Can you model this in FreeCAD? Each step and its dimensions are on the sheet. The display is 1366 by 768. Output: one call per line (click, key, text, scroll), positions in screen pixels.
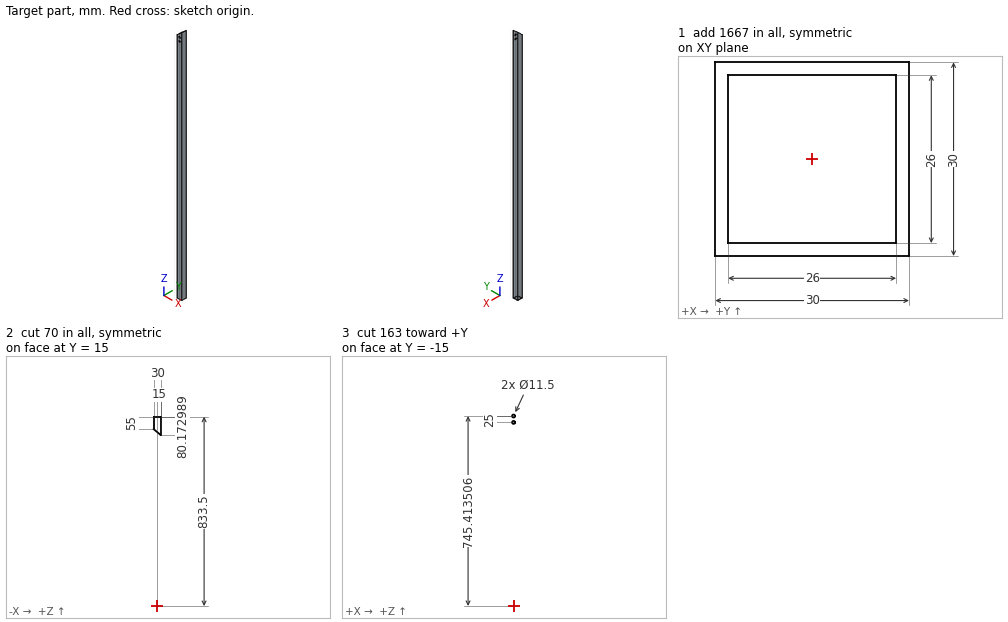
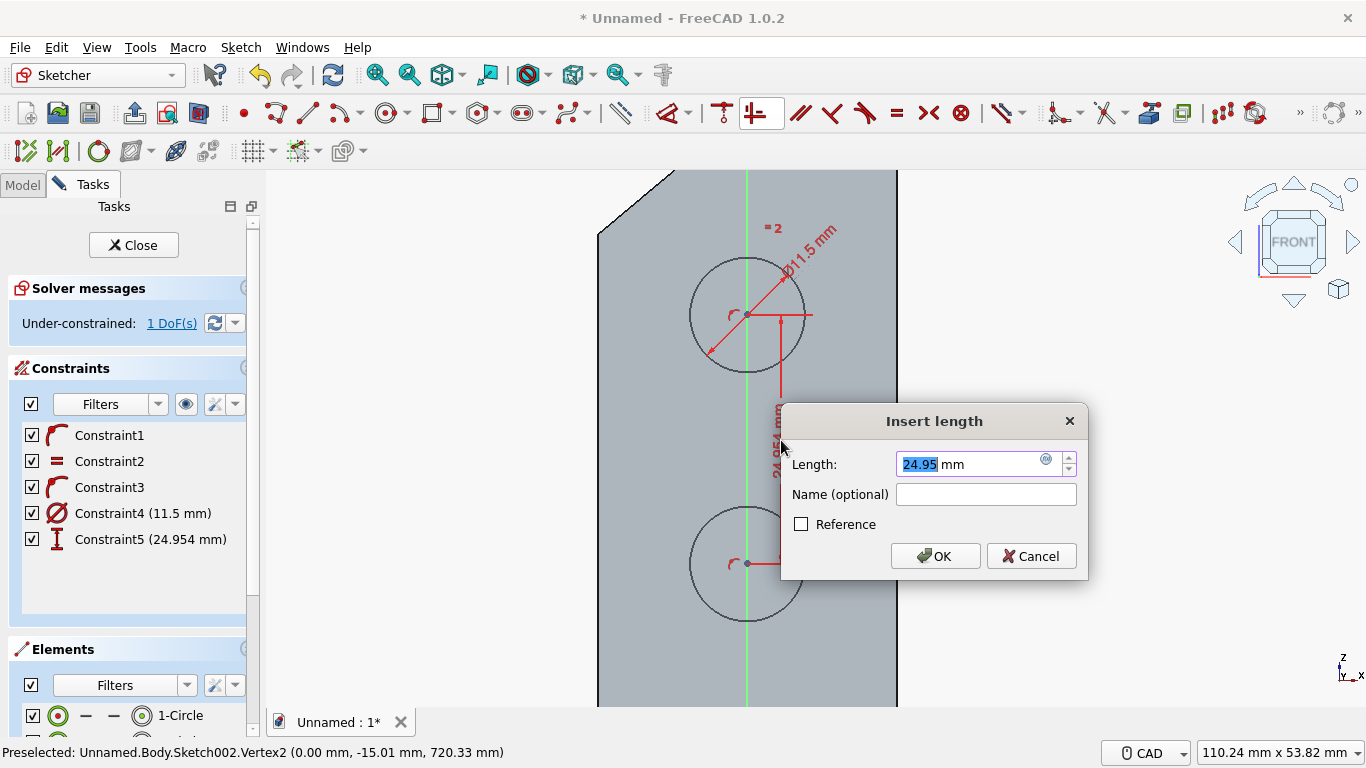
text(25)
key(Return)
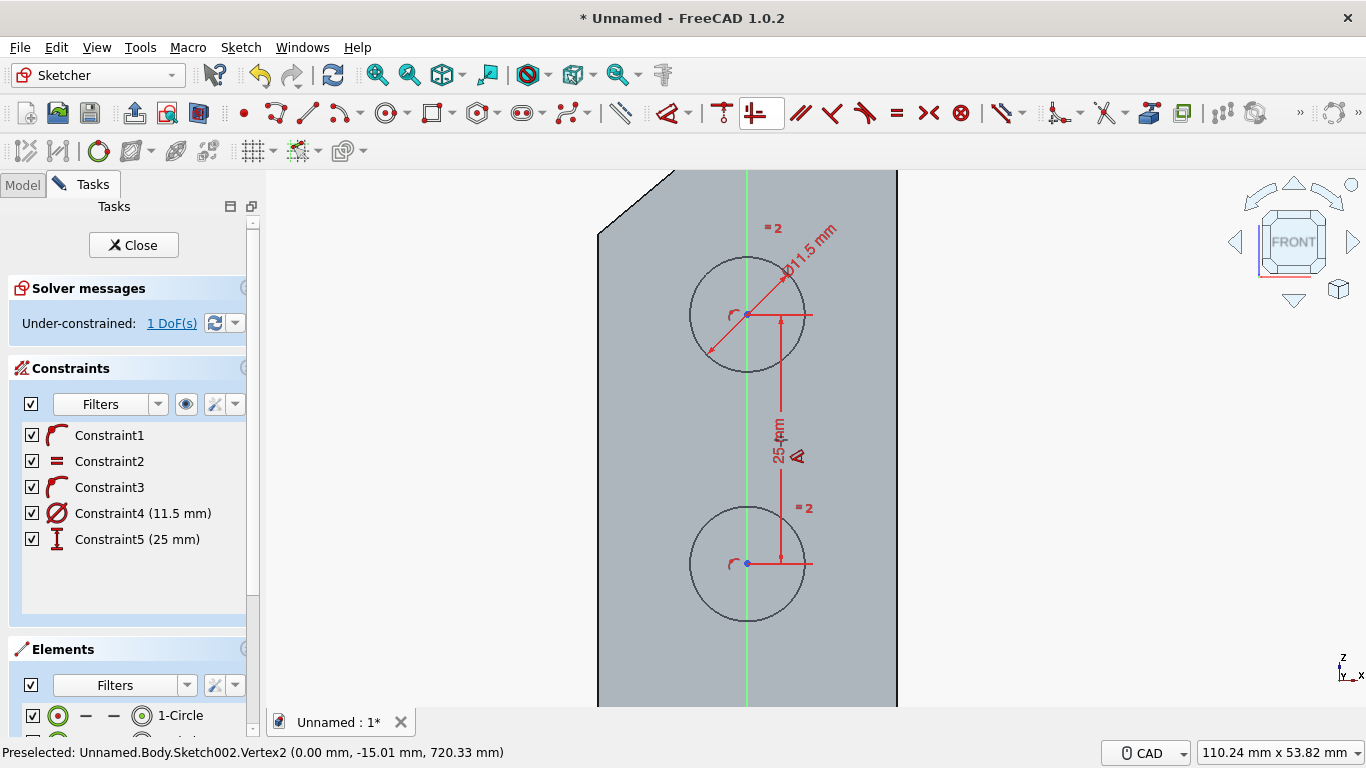
click(747, 315)
click(781, 497)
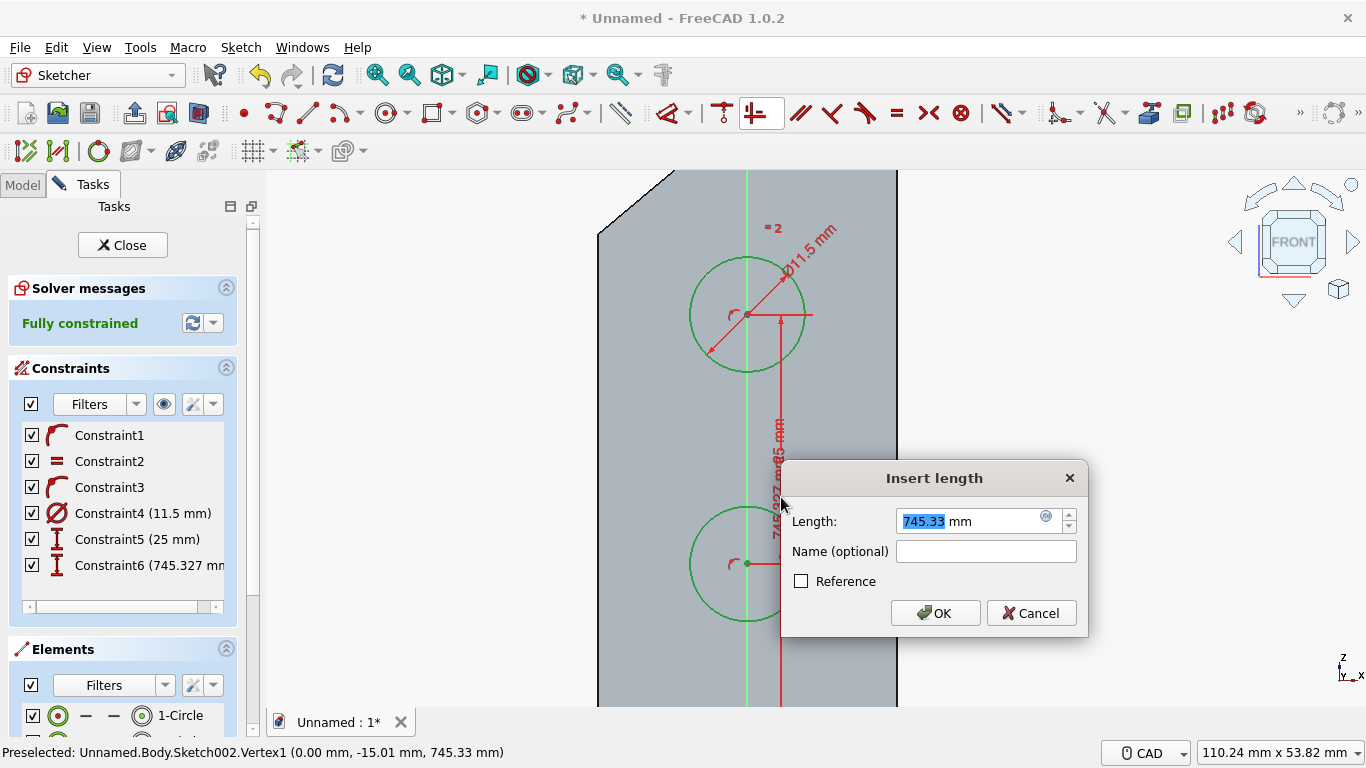
text(745.413506)
key(Return)
key(Escape)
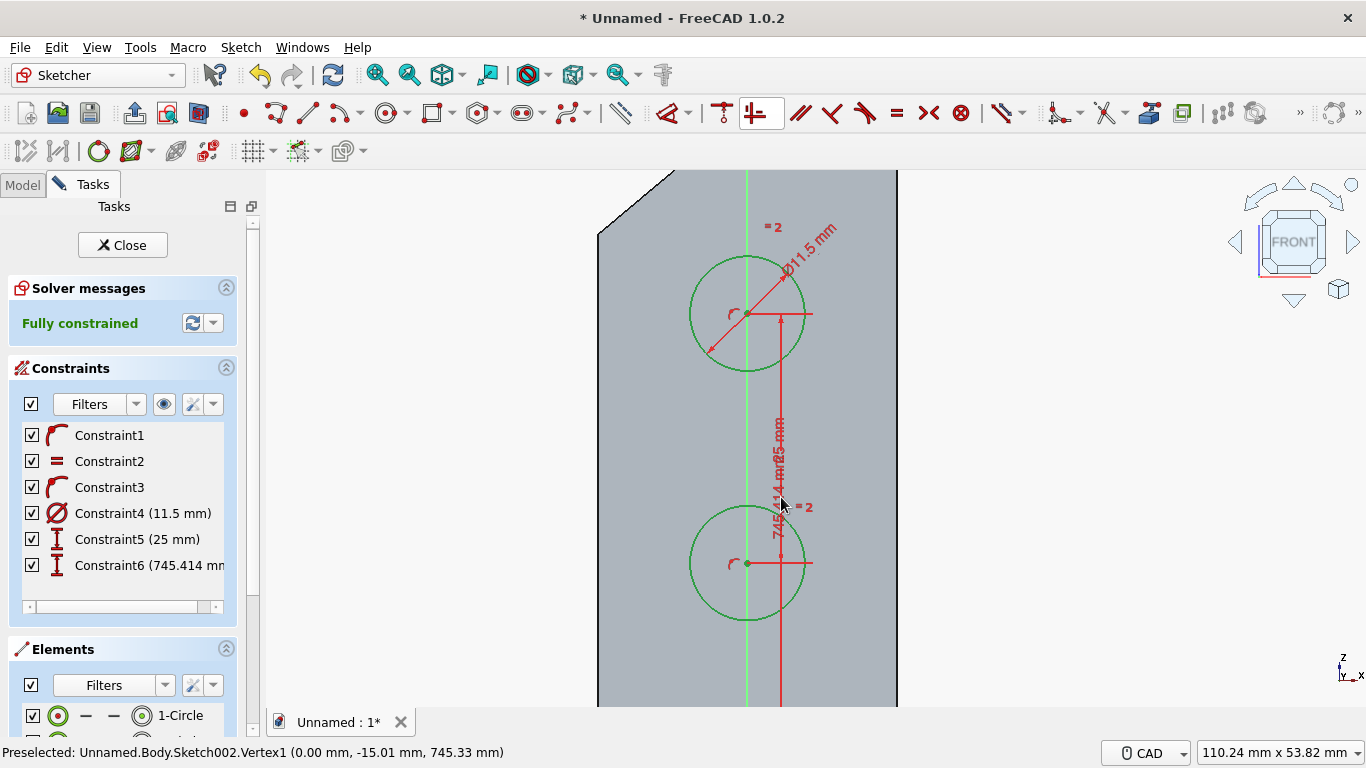
click(123, 245)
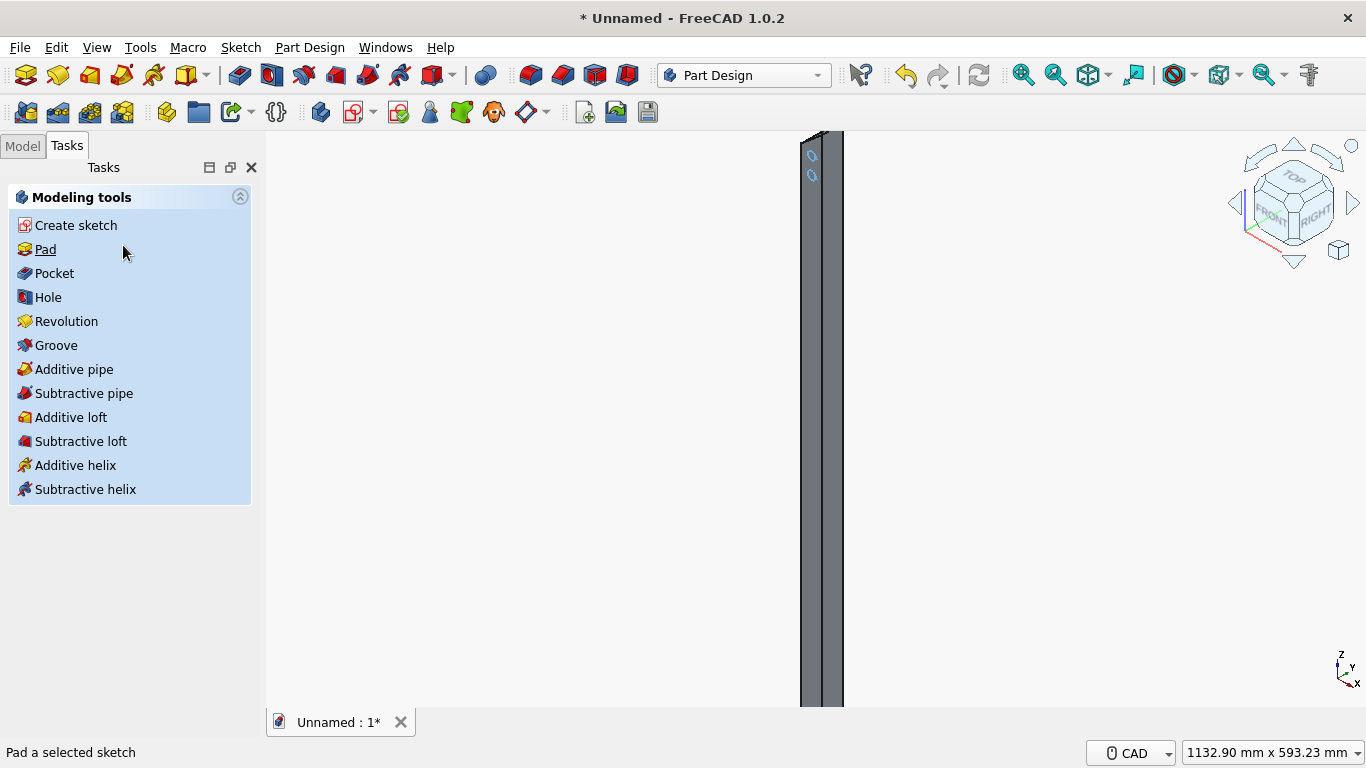
click(240, 76)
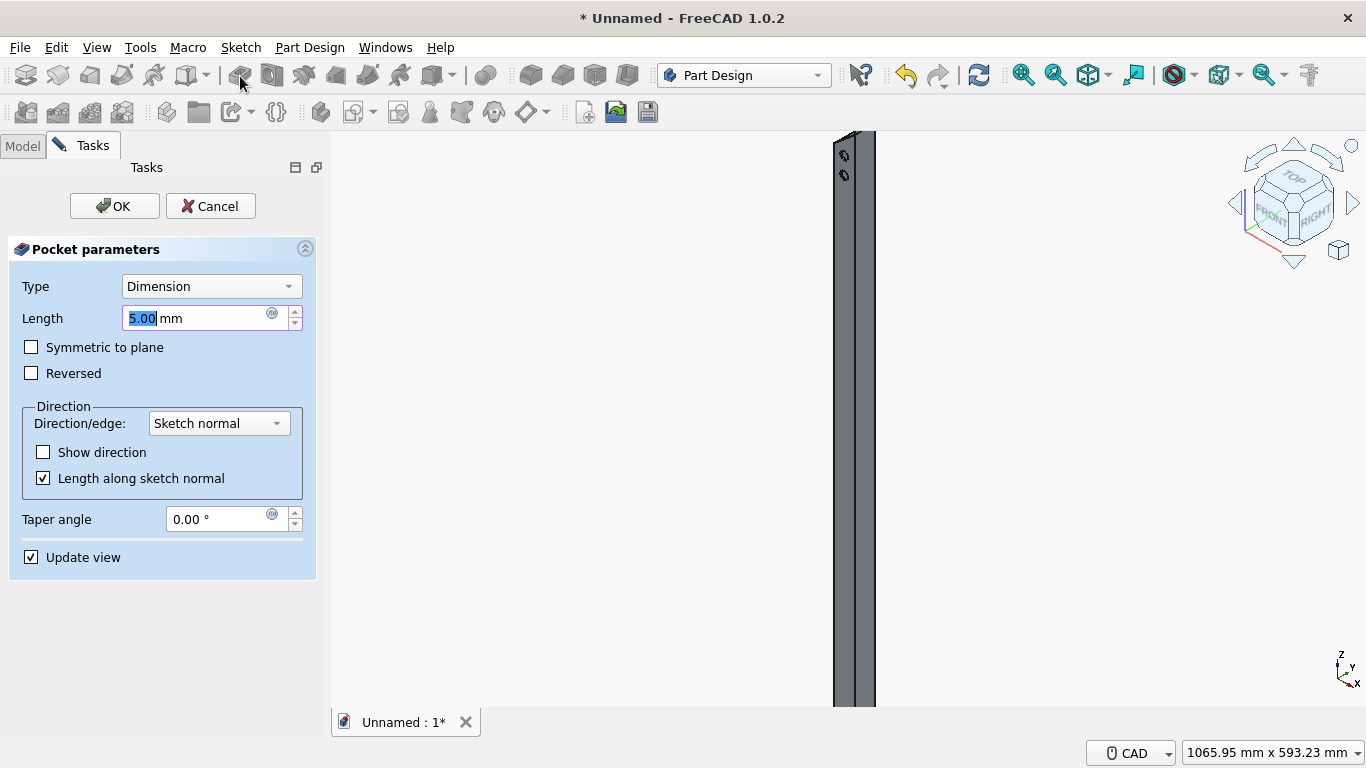
text(163)
key(Tab)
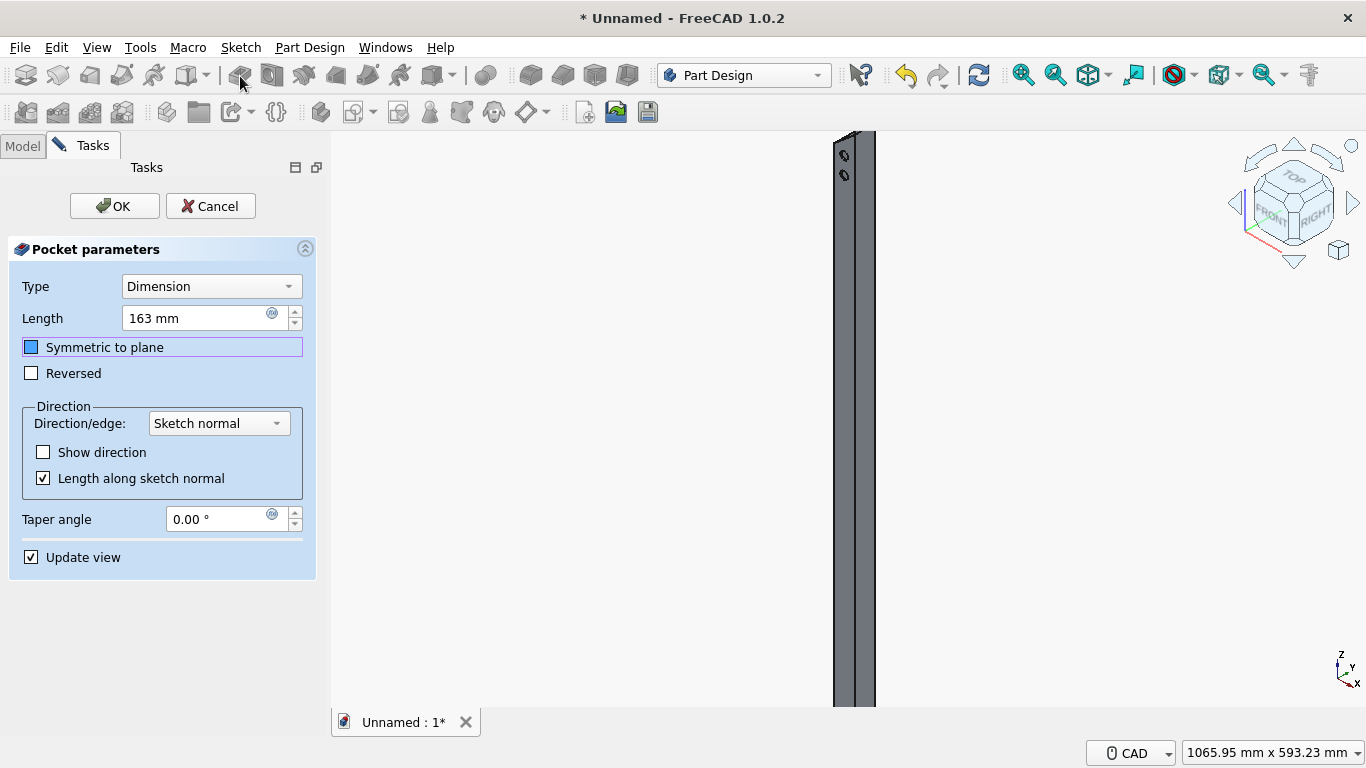
click(115, 206)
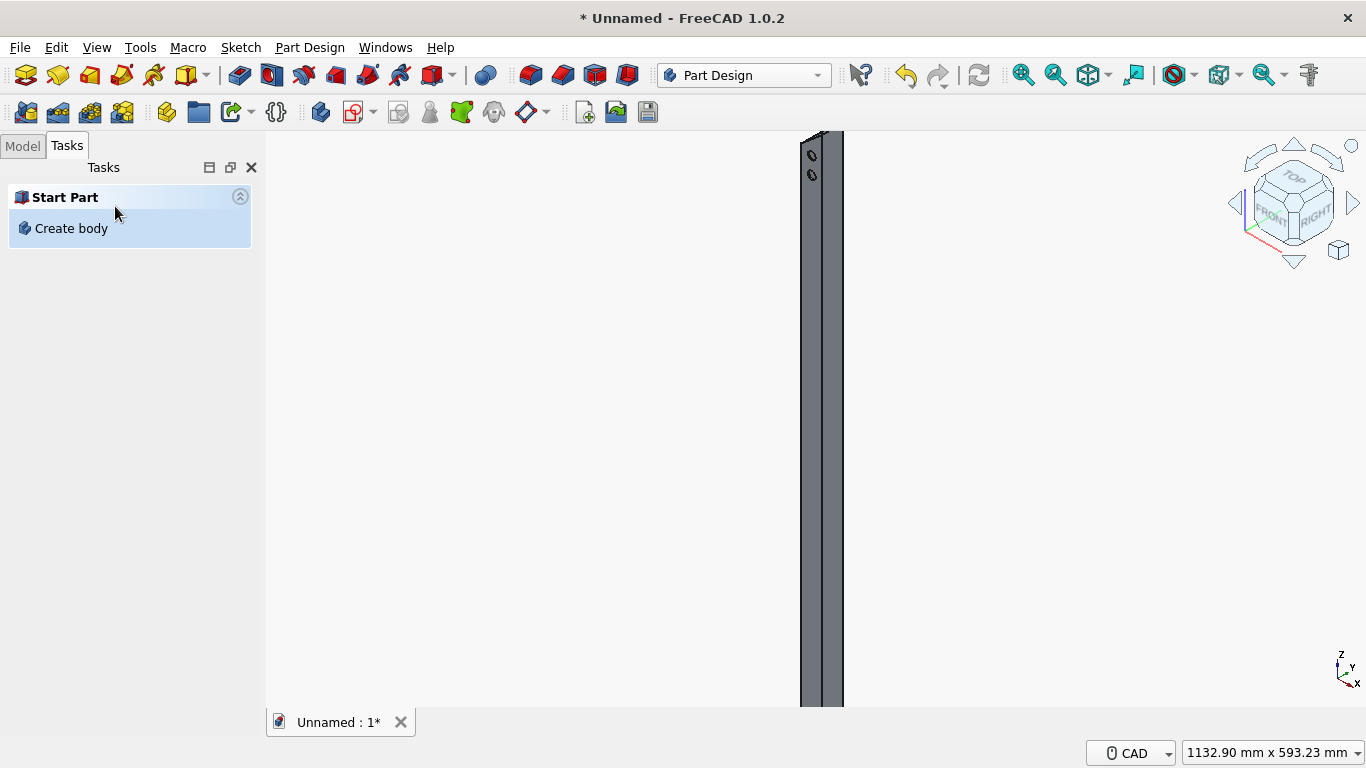
click(1024, 76)